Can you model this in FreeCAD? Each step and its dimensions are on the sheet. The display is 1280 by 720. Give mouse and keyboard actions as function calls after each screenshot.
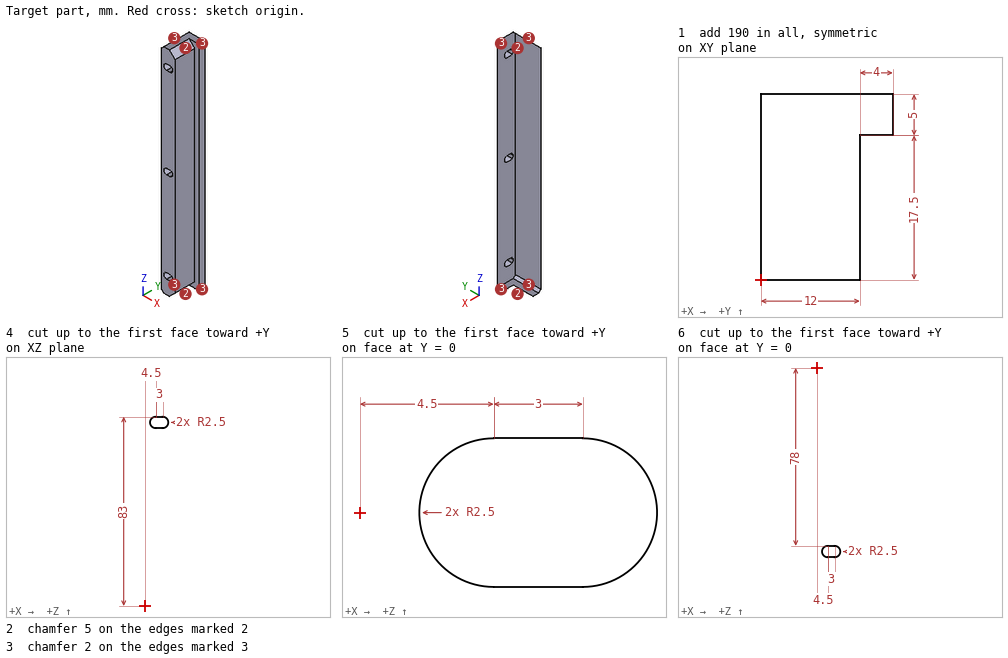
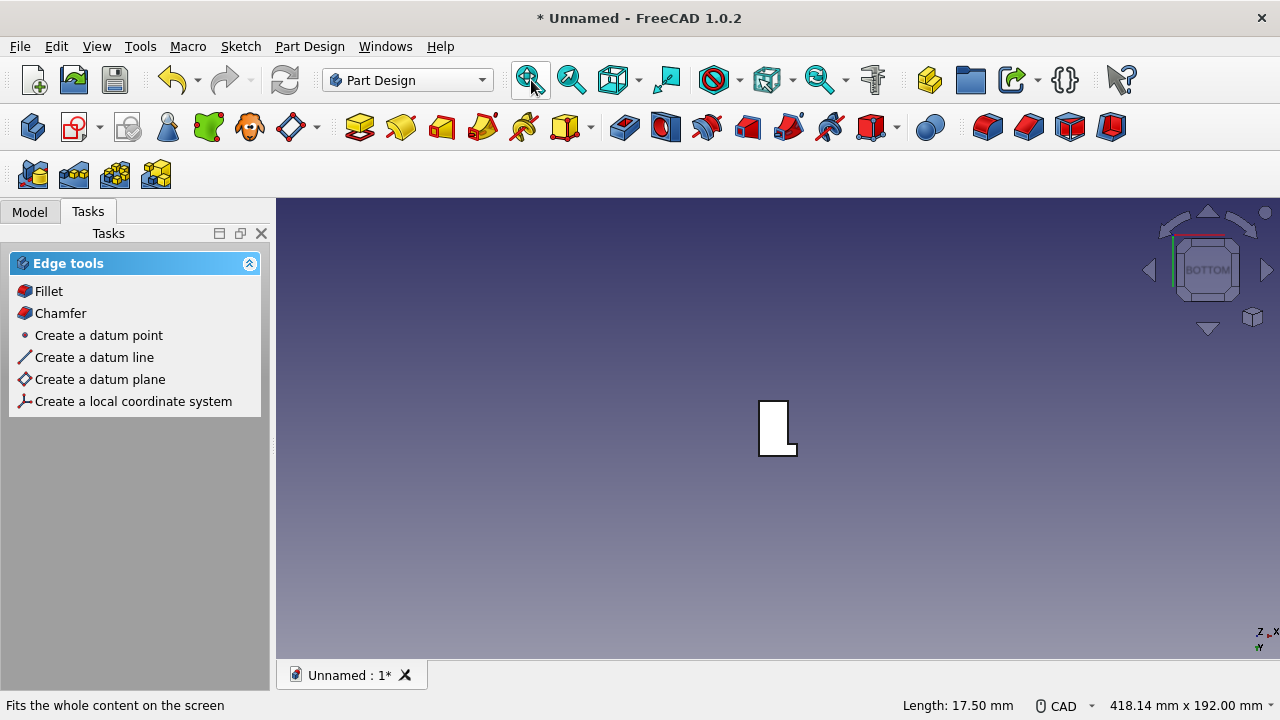
click(788, 421, ctrl)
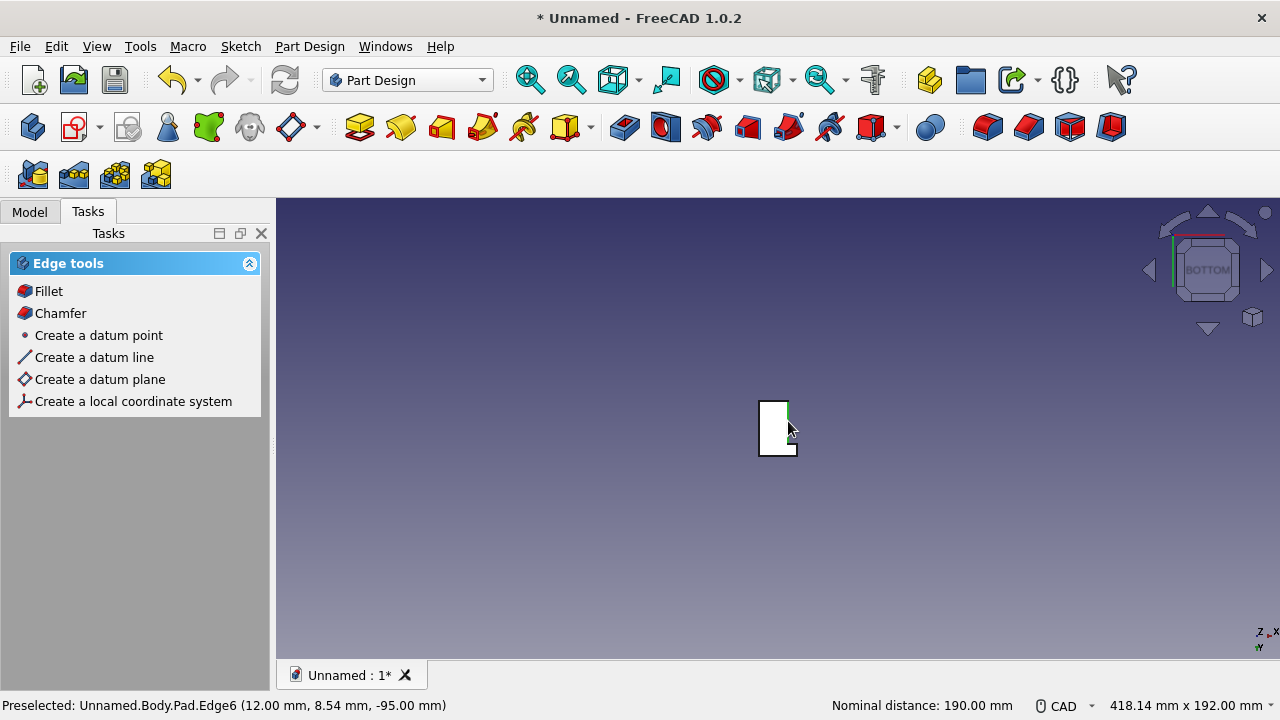
click(1029, 128)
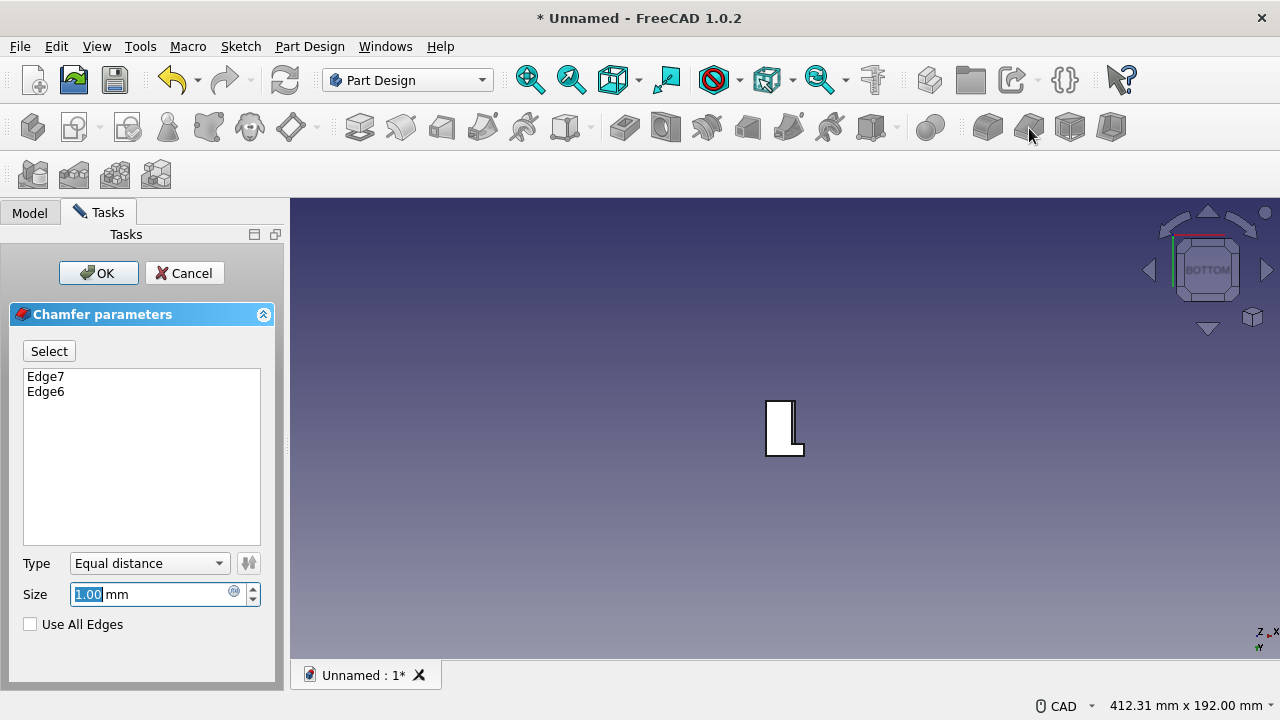
text(5)
key(Tab)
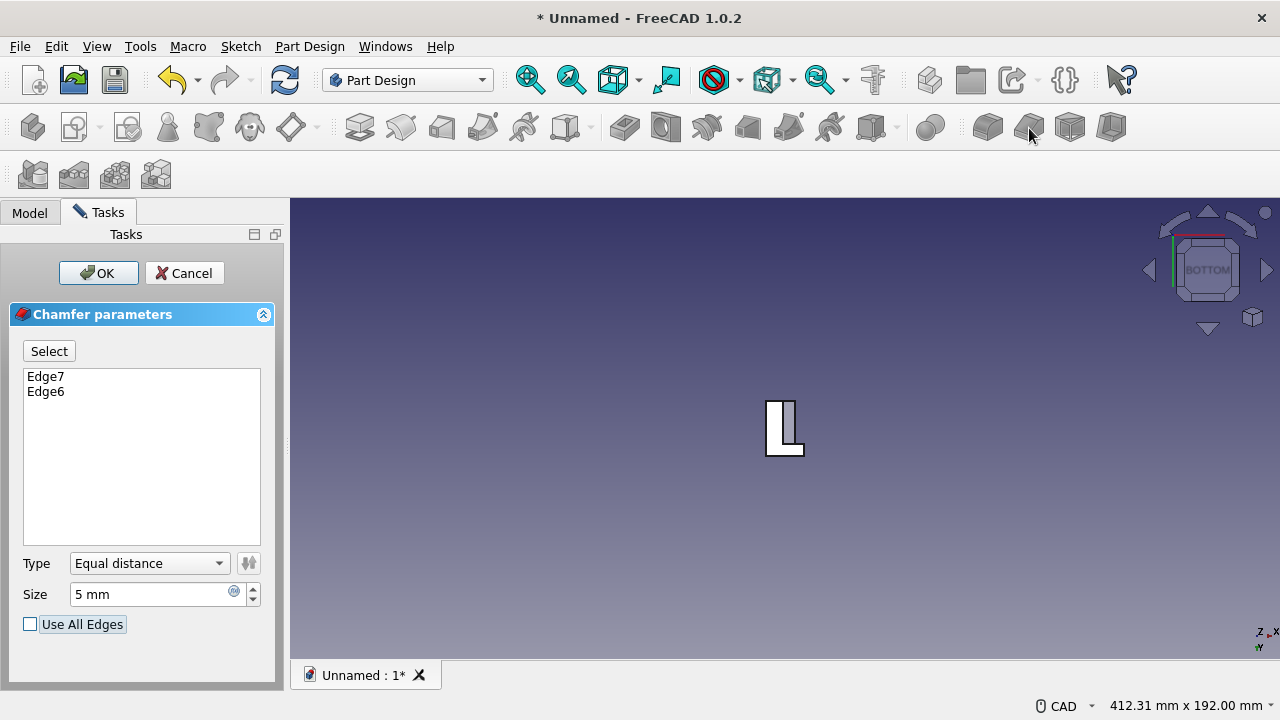
click(99, 273)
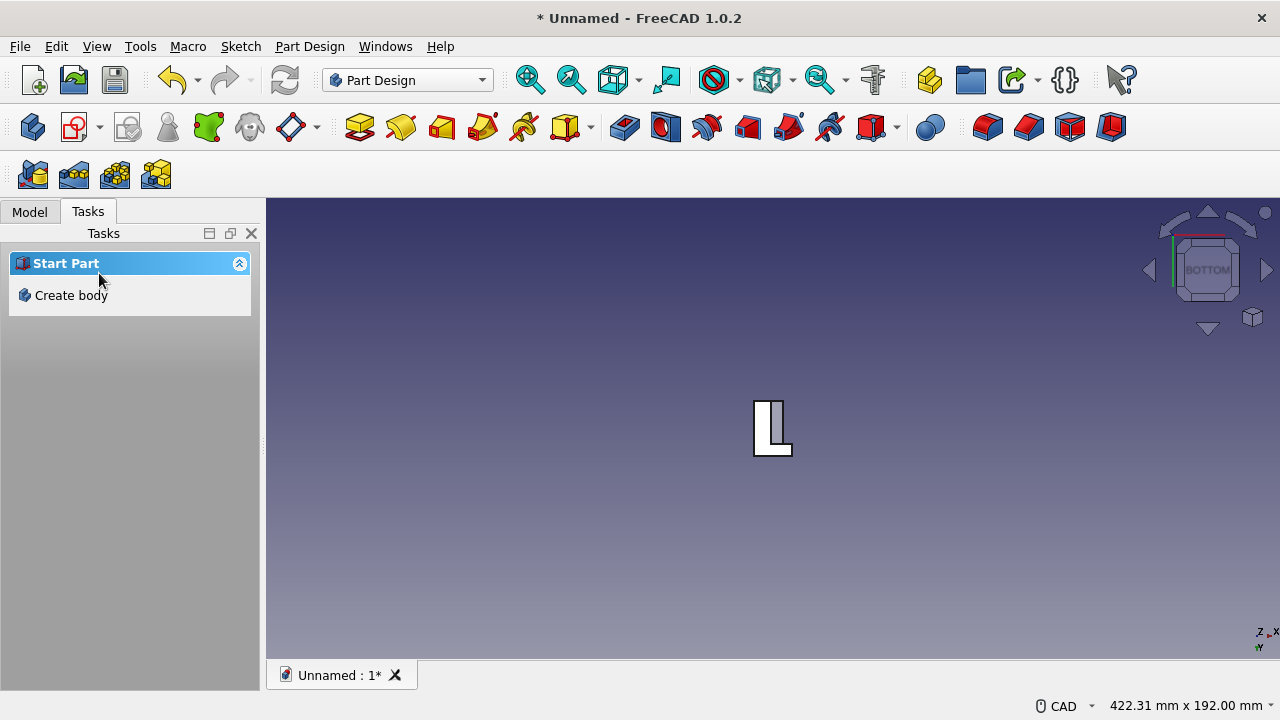
click(531, 80)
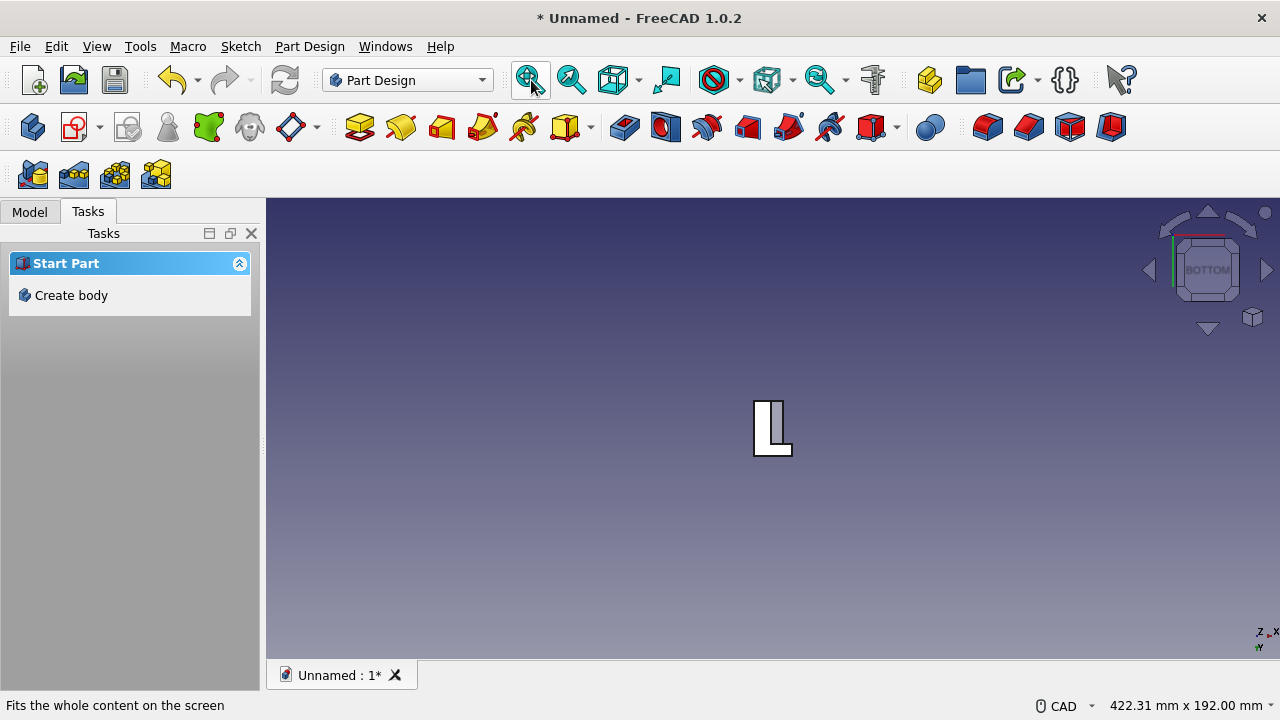
click(754, 427)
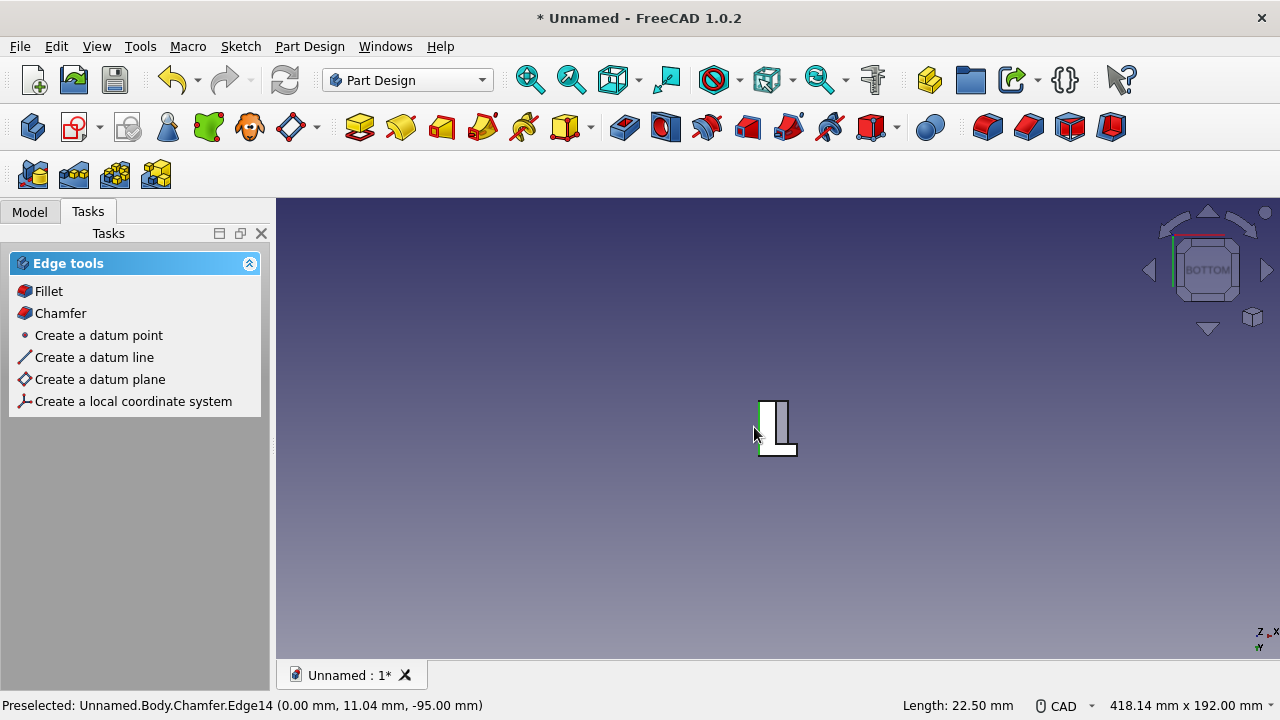
scroll(797, 449, up, 7)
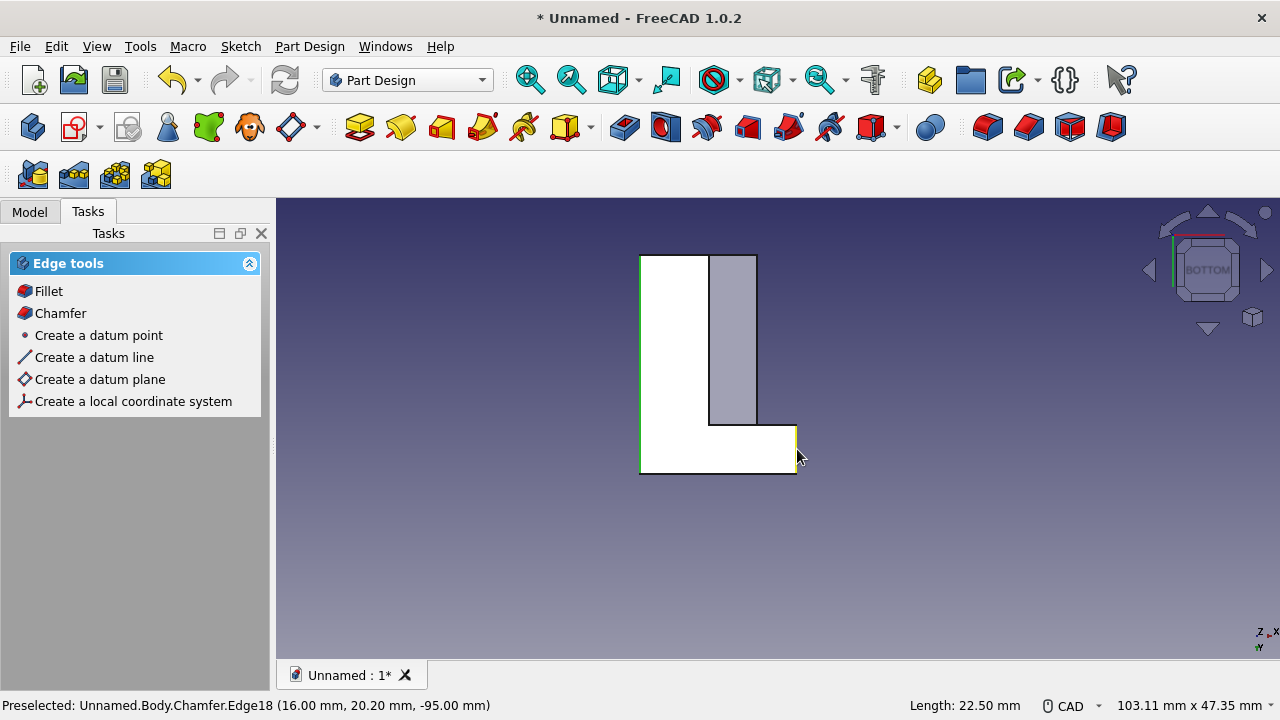
click(796, 448, ctrl)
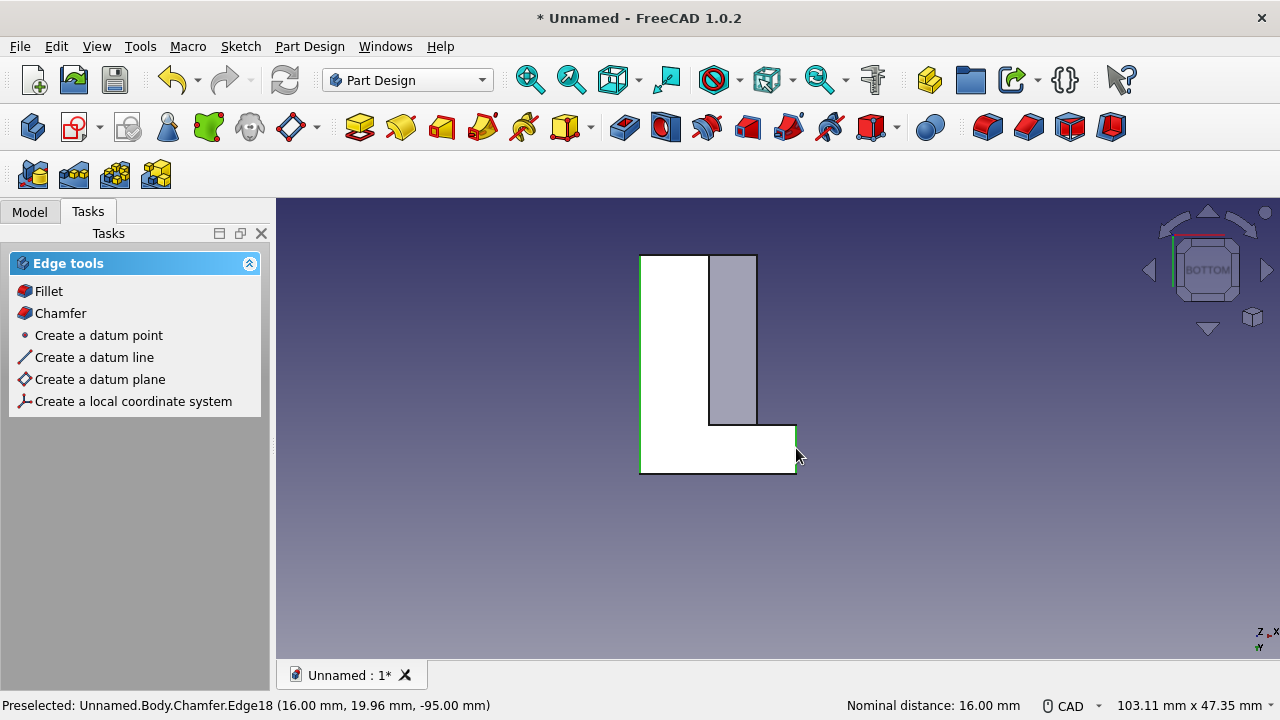
click(531, 80)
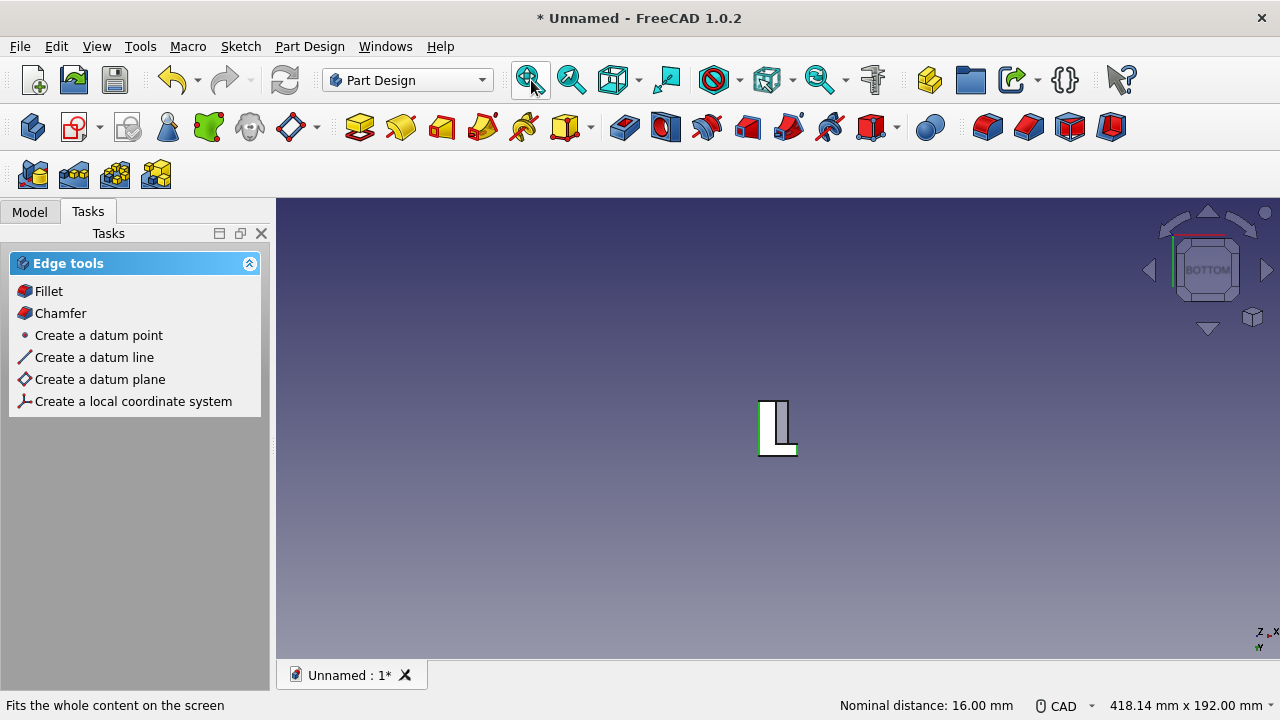
key(0)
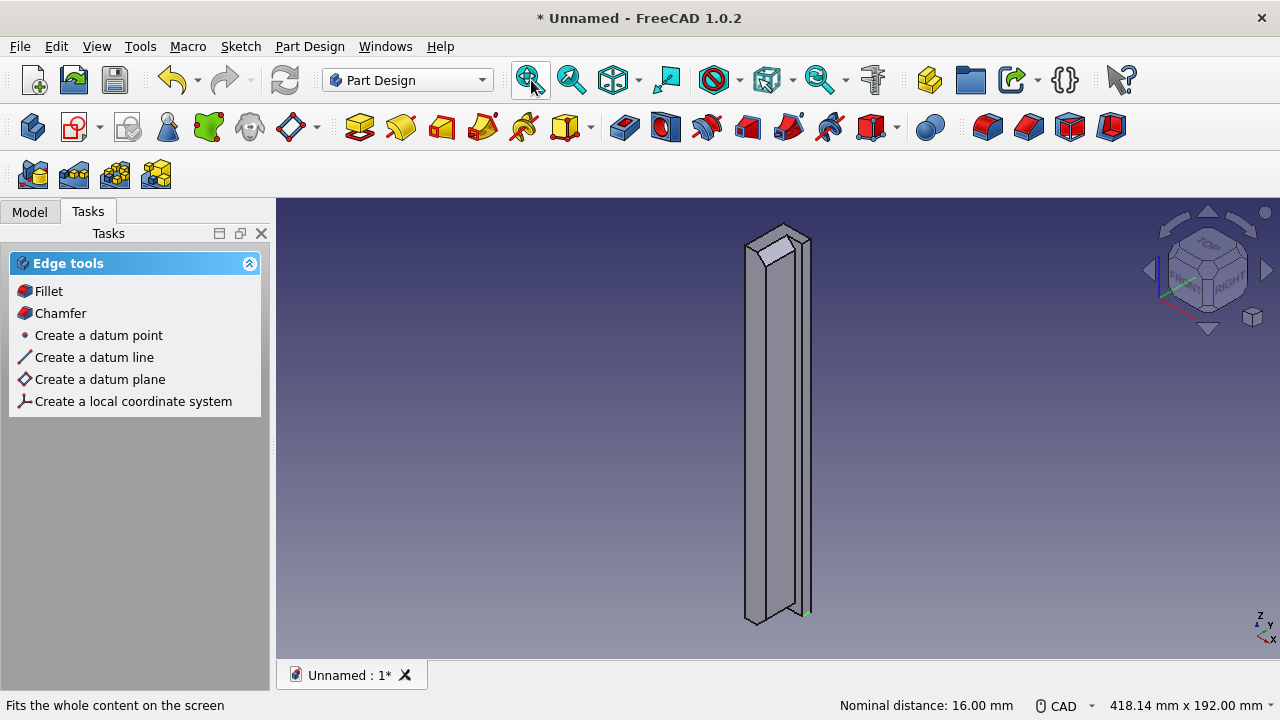
click(808, 240, ctrl)